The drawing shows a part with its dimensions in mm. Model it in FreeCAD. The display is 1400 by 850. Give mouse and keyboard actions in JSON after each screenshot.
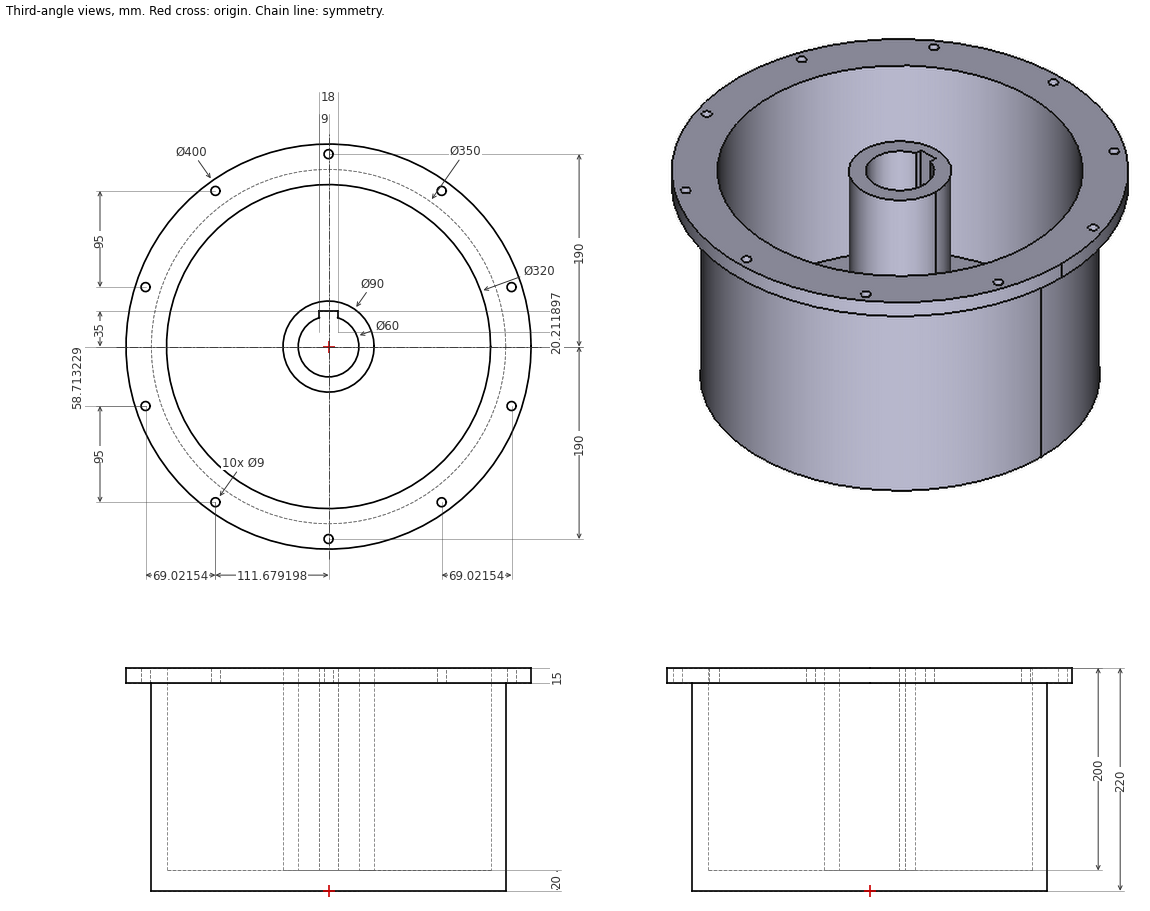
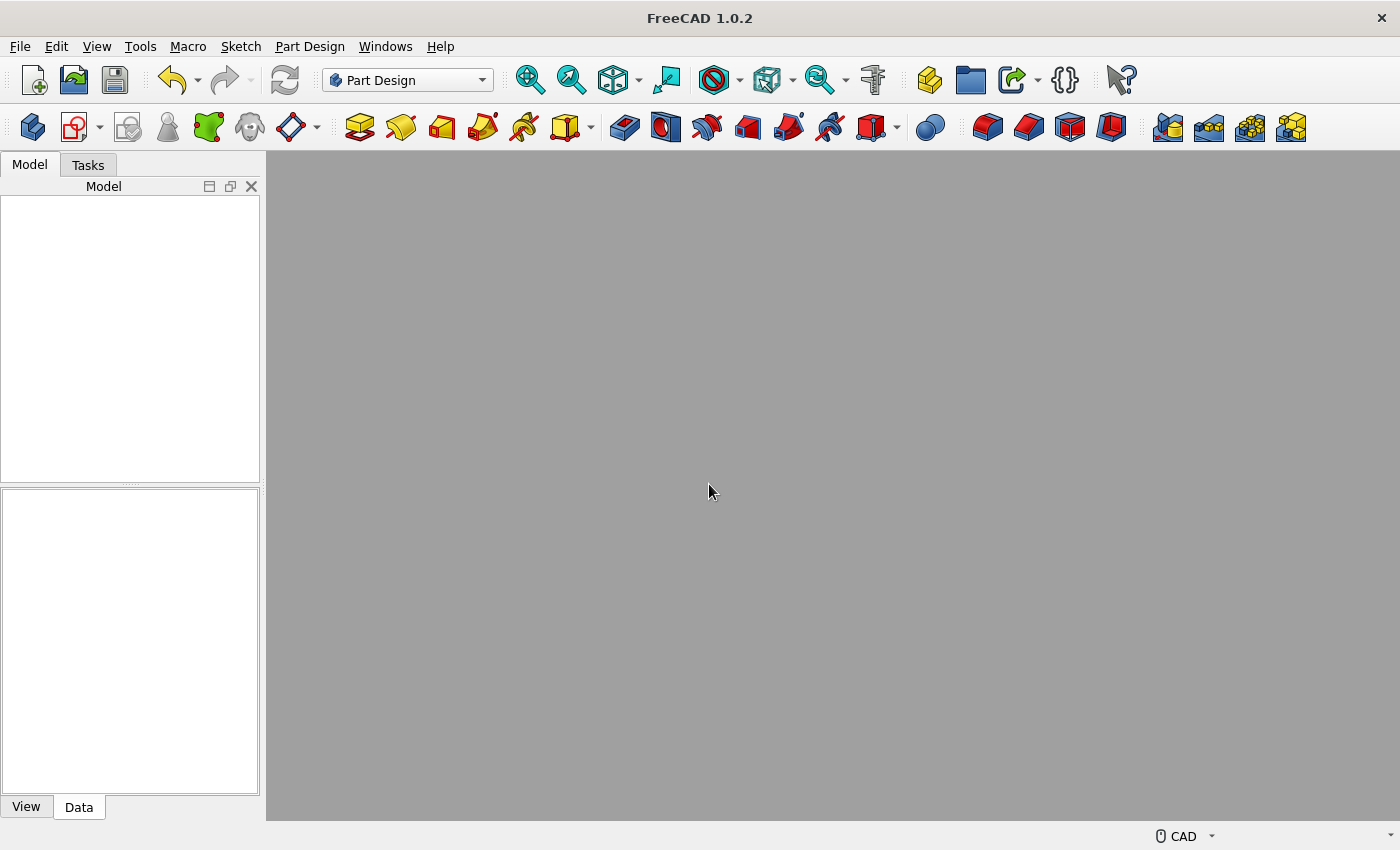
{"action": "left_click", "coordinate": [33, 80]}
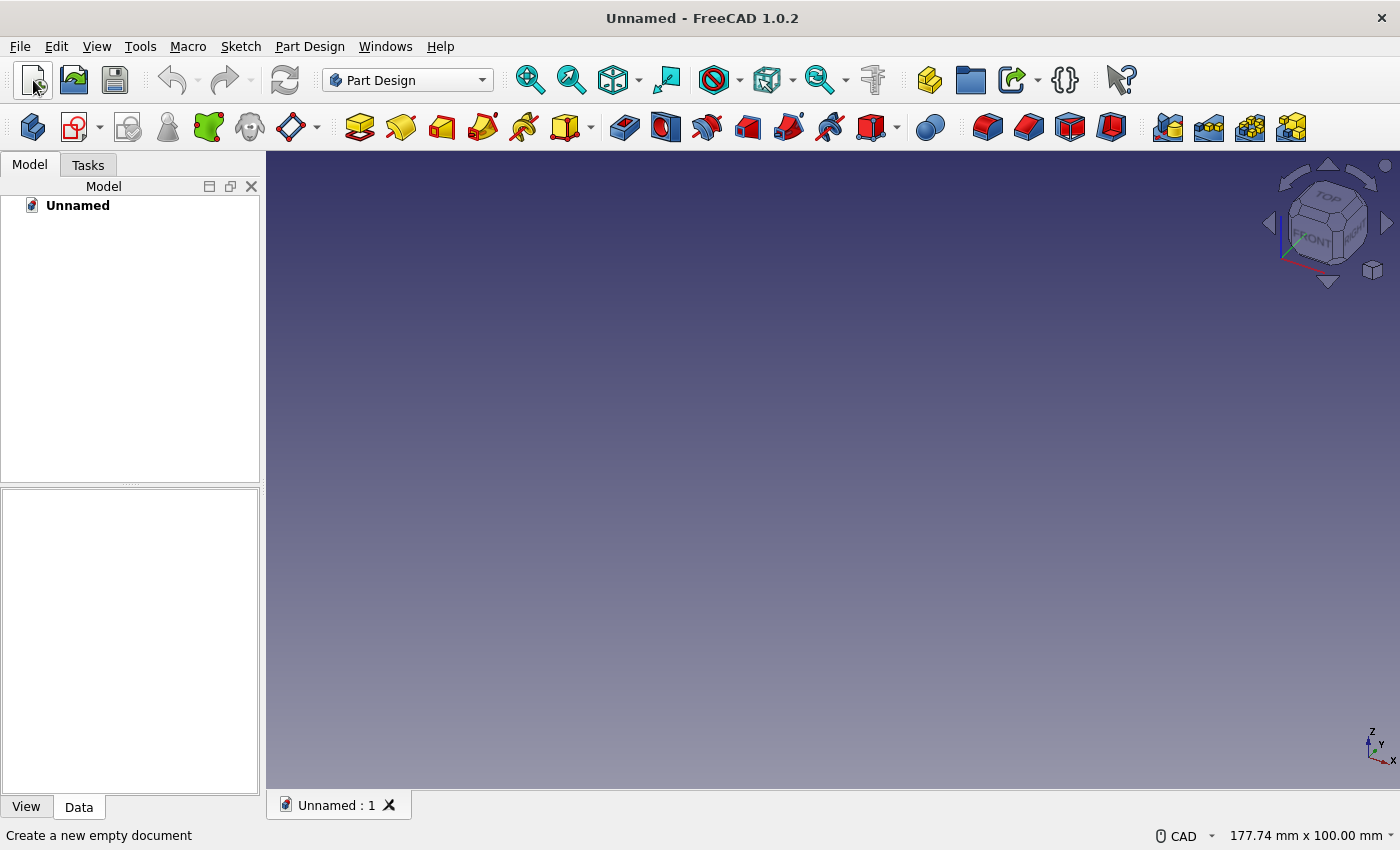
{"action": "left_click", "coordinate": [74, 128]}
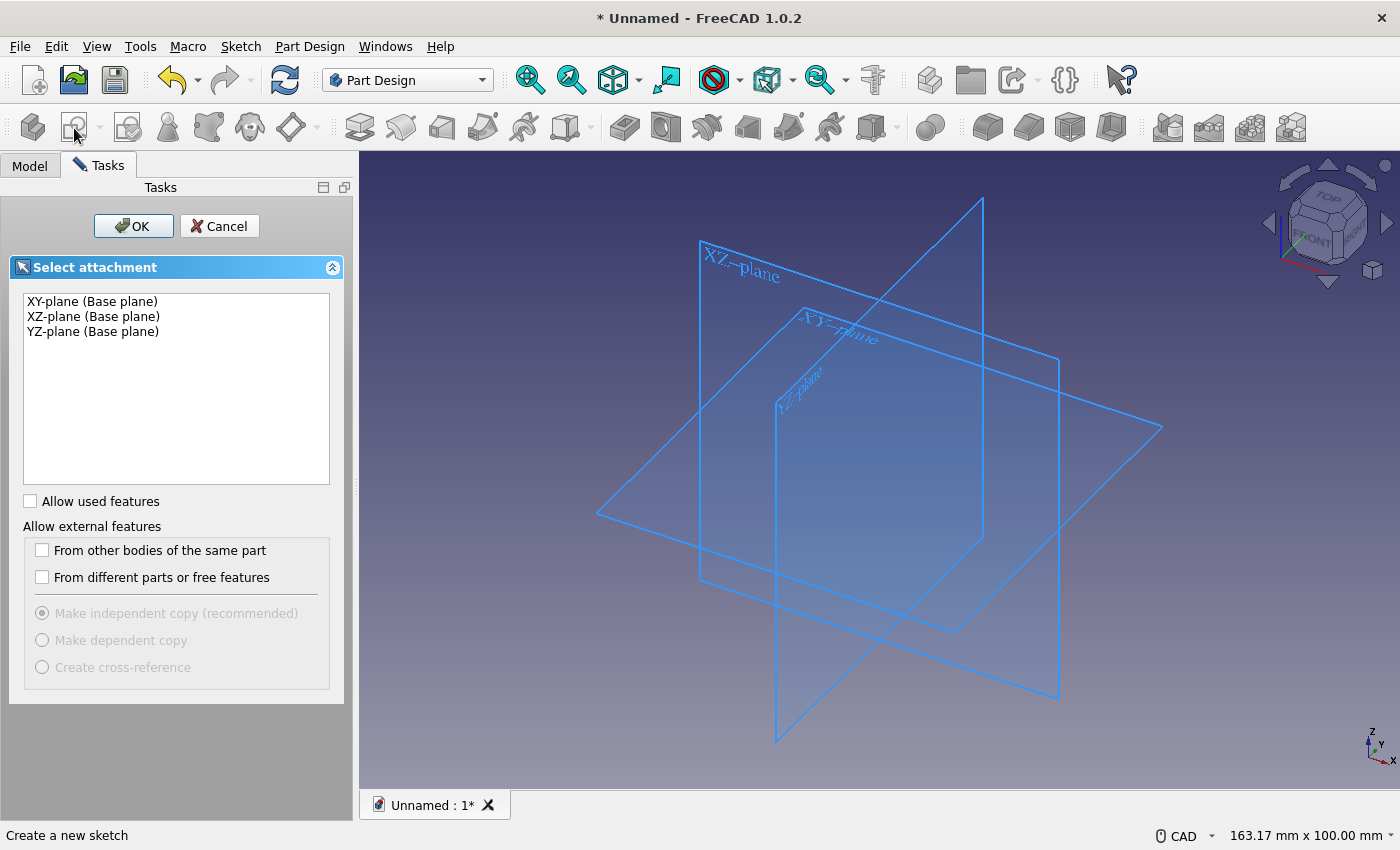
{"action": "left_click", "coordinate": [84, 302]}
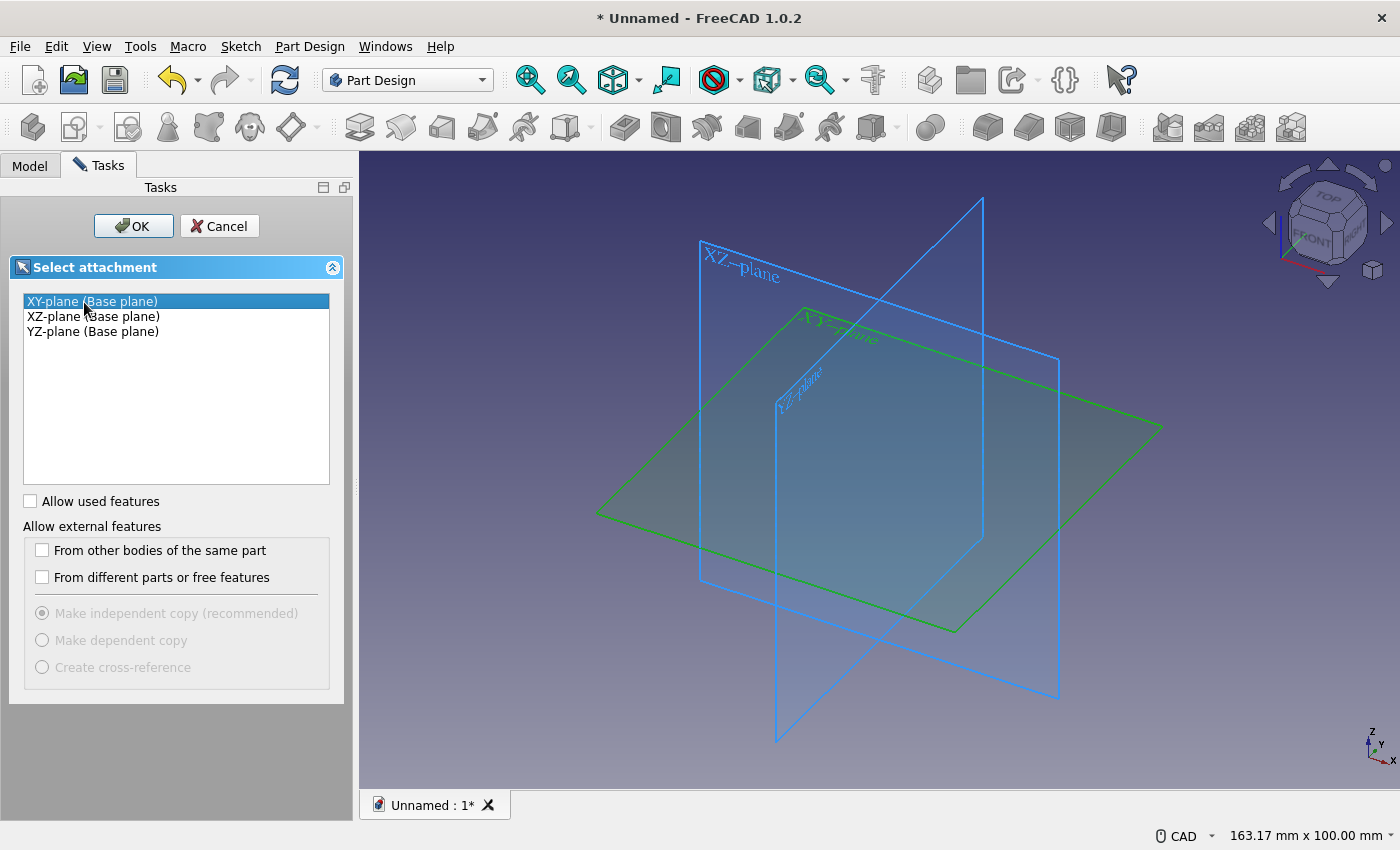
{"action": "left_click", "coordinate": [134, 226]}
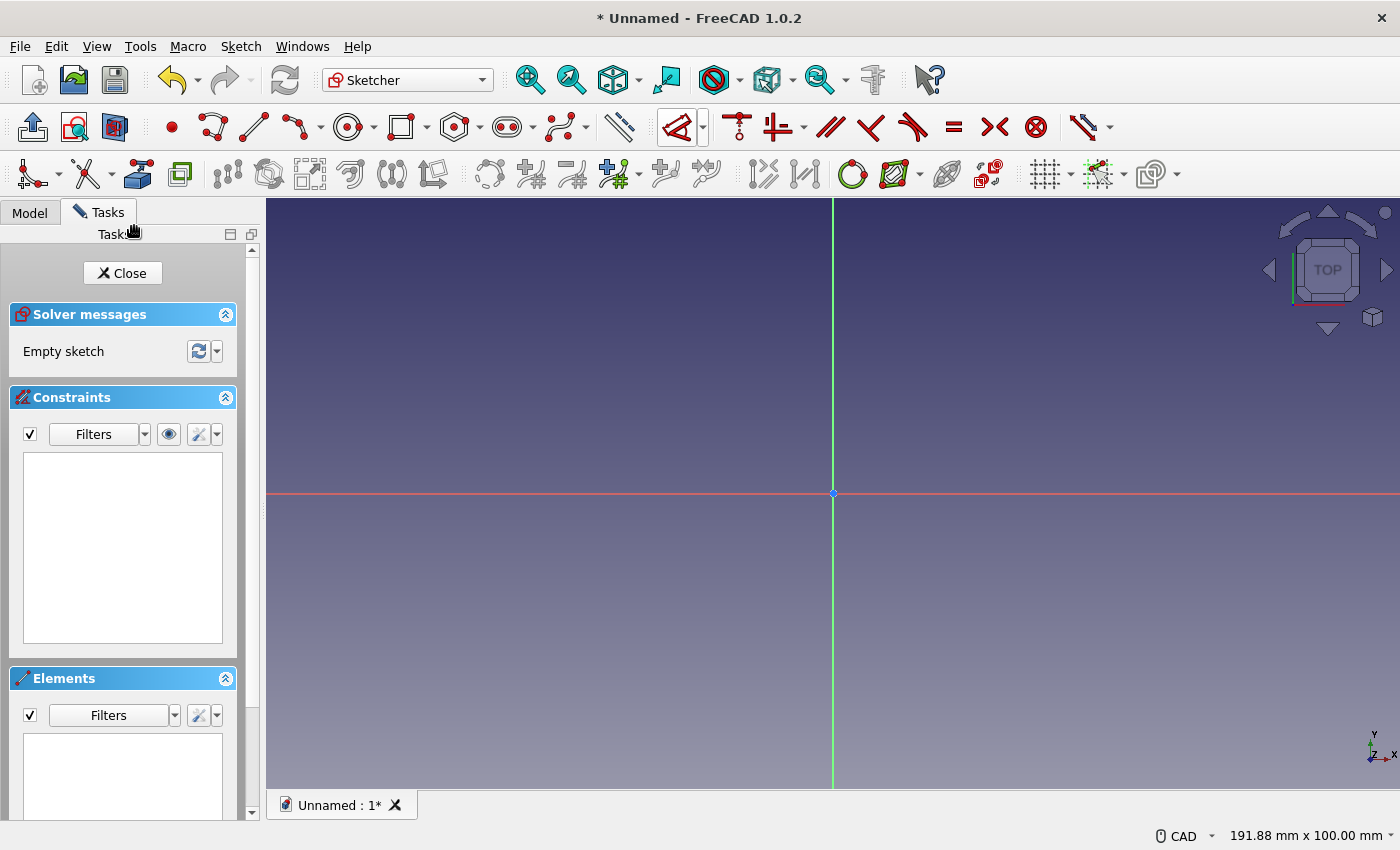
{"action": "scroll", "coordinate": [751, 494], "scroll_direction": "down", "scroll_amount": 9}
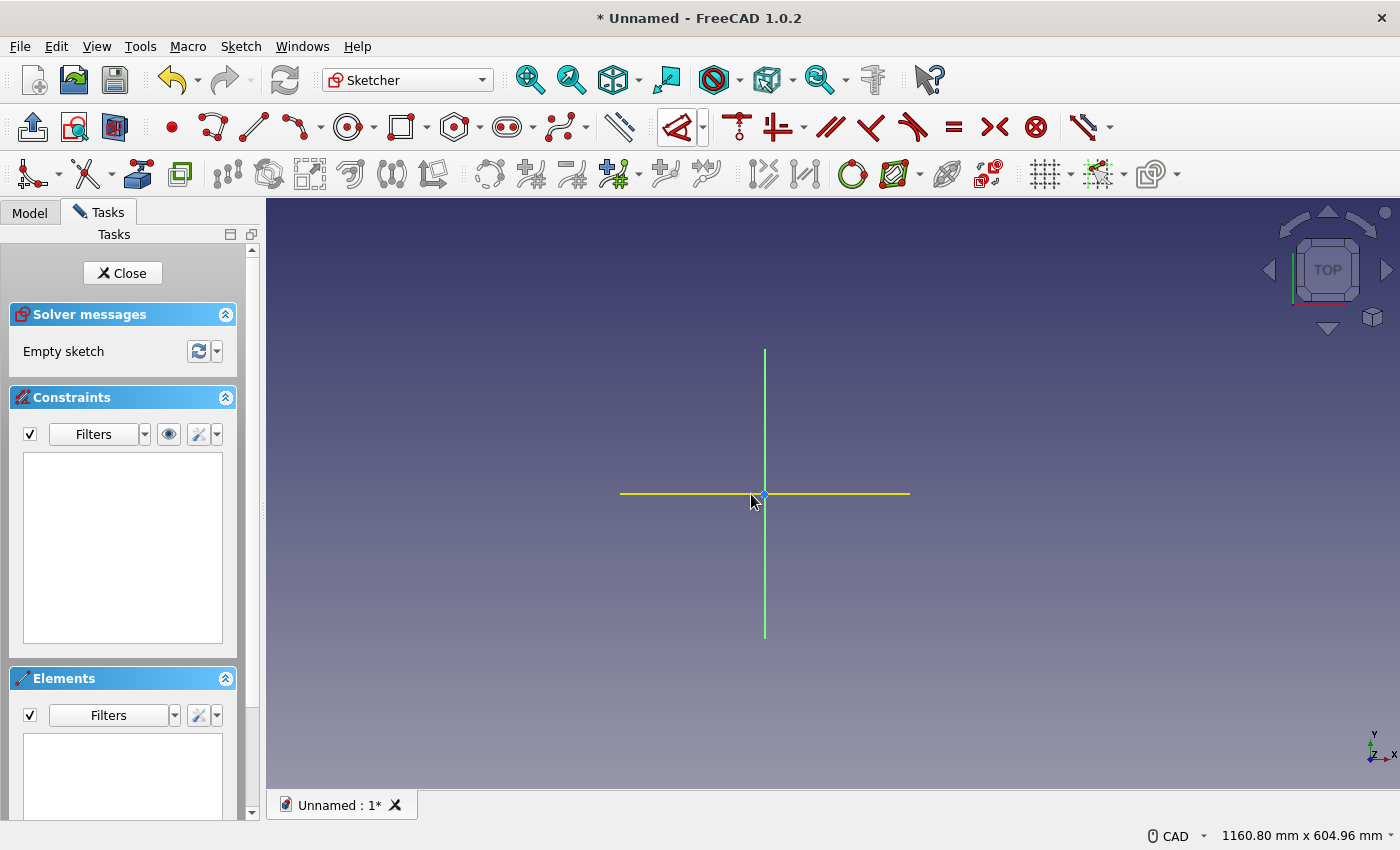
{"action": "left_click", "coordinate": [348, 128]}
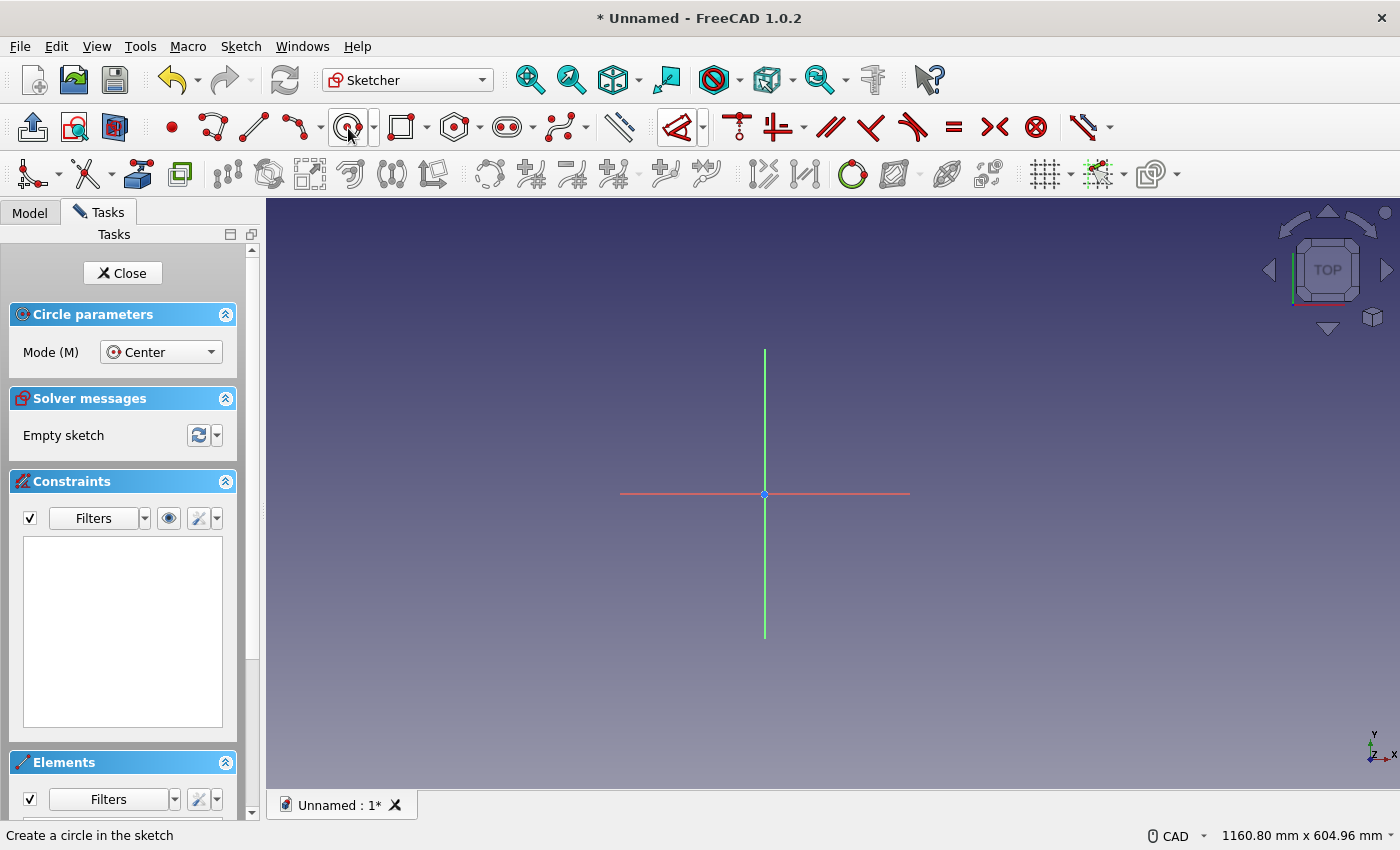
{"action": "left_click", "coordinate": [765, 494]}
{"action": "mouse_move", "coordinate": [886, 373]}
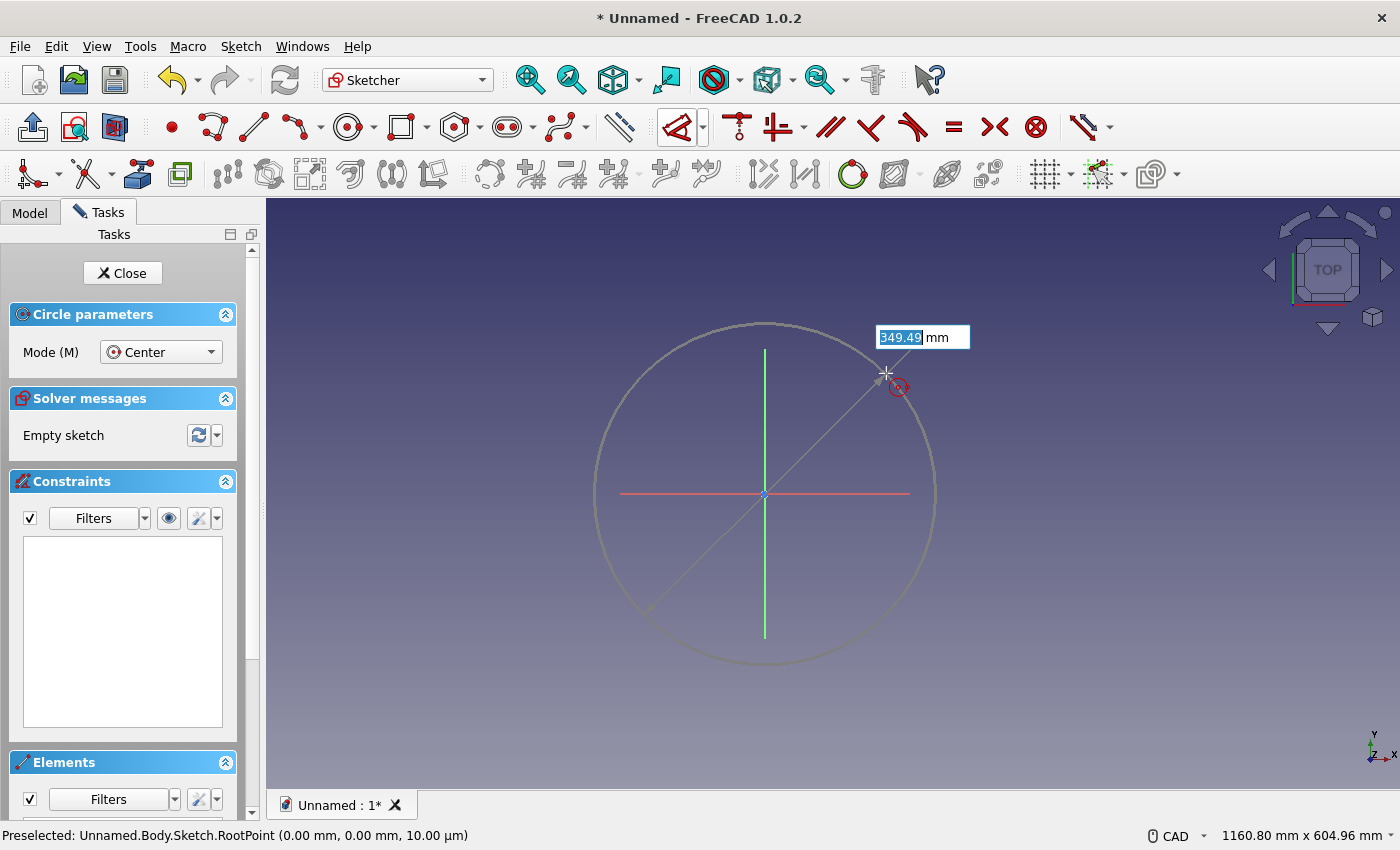
{"action": "type", "text": "350"}
{"action": "key", "text": "Return"}